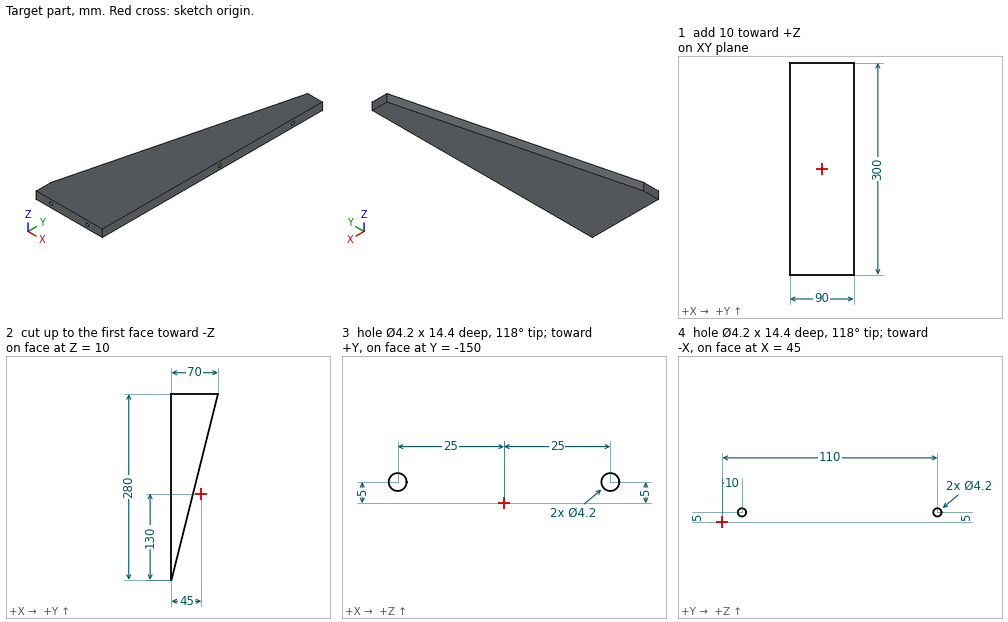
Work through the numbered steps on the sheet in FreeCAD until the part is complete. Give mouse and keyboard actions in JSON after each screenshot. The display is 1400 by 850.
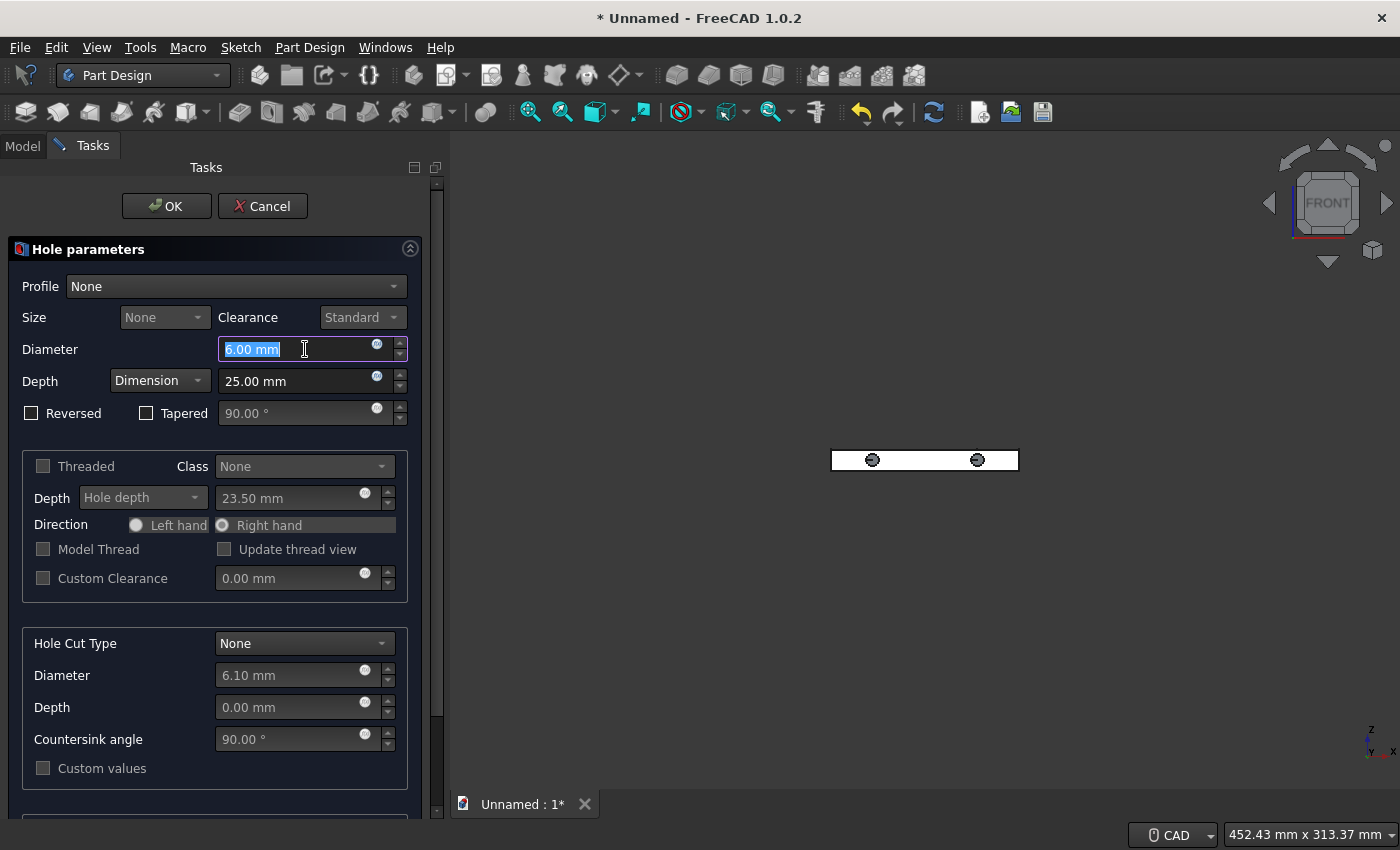
{"action": "type", "text": "4.2"}
{"action": "key", "text": "Tab"}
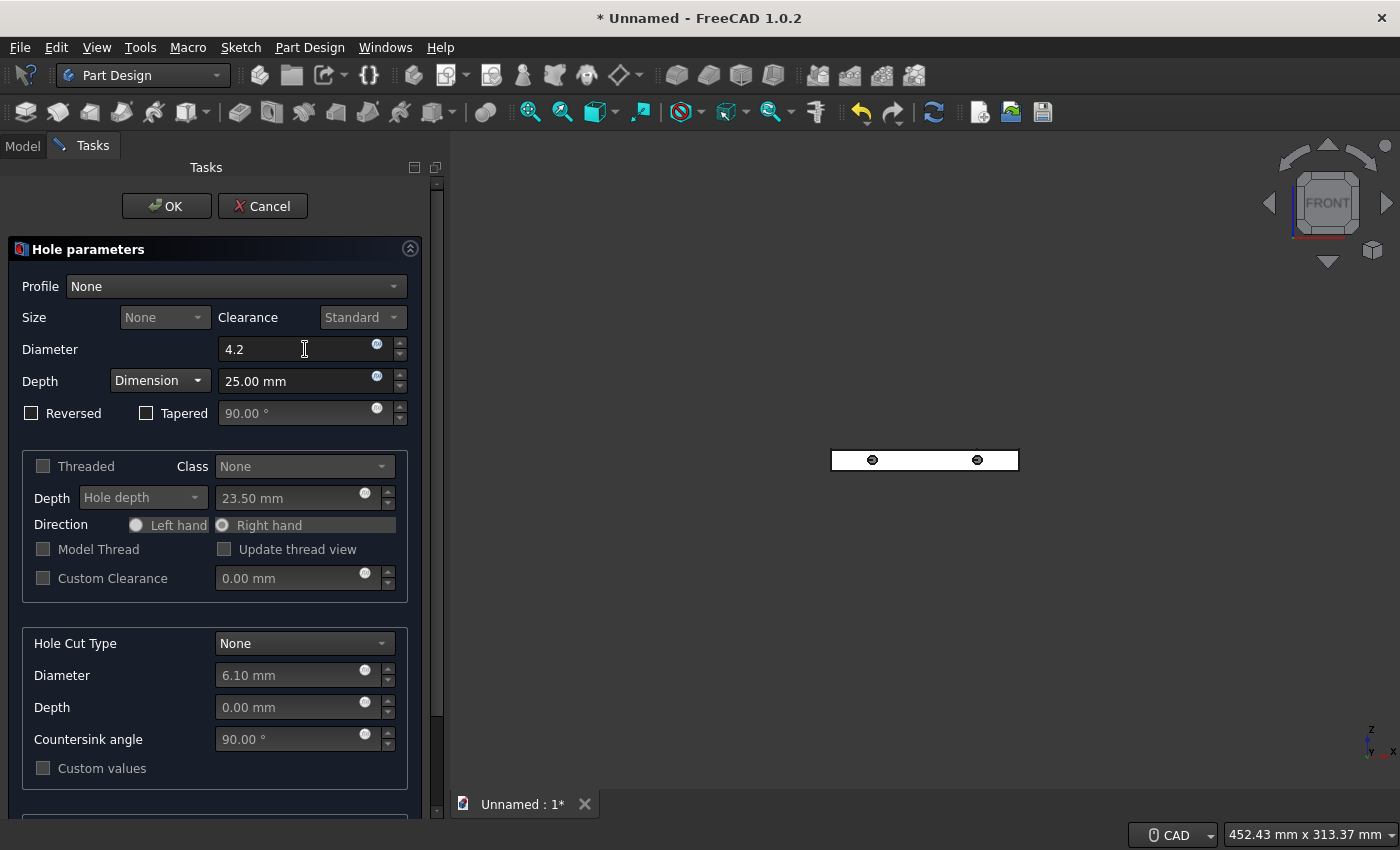
{"action": "triple_click", "coordinate": [305, 381]}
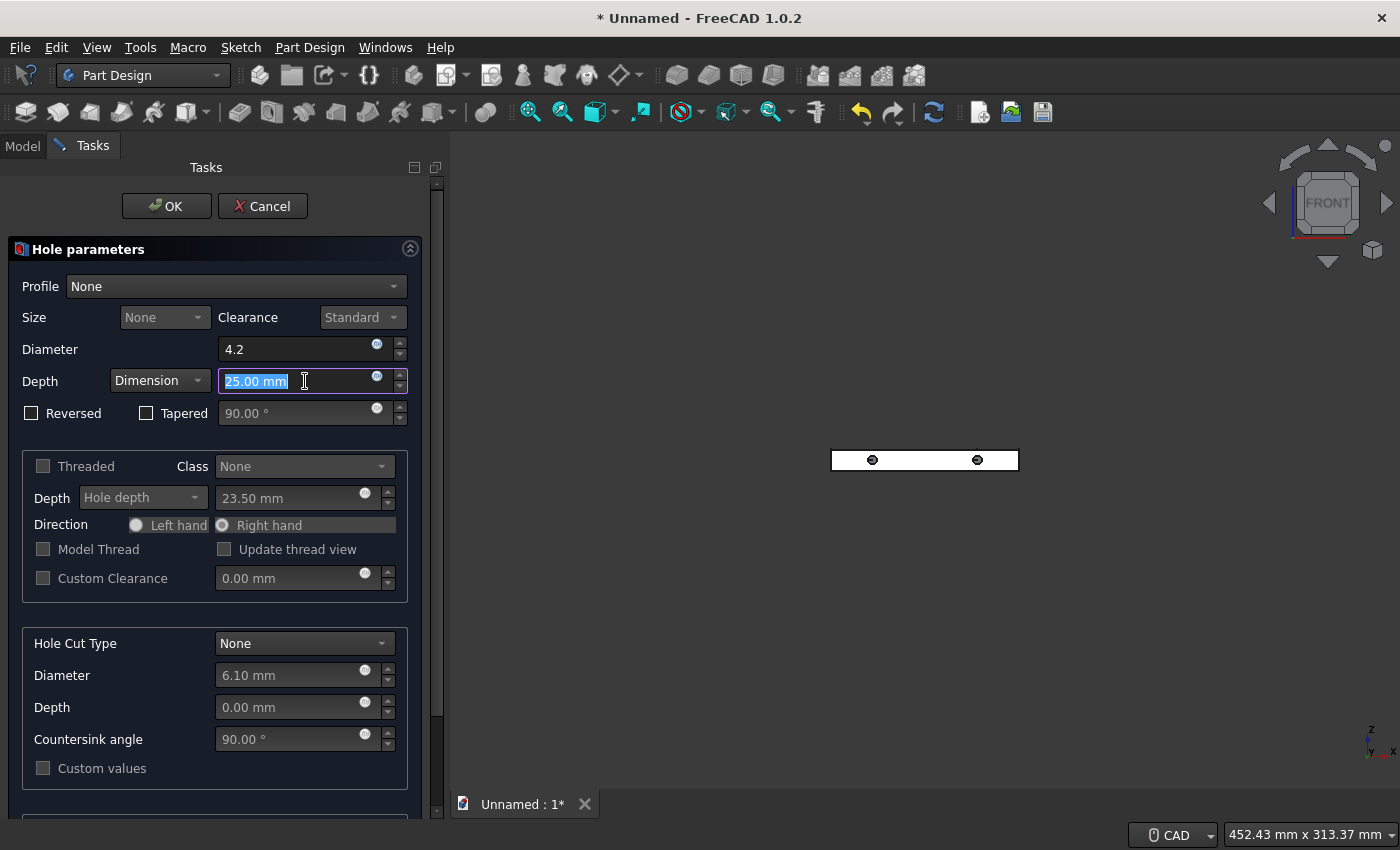
{"action": "type", "text": "14.4"}
{"action": "key", "text": "Tab"}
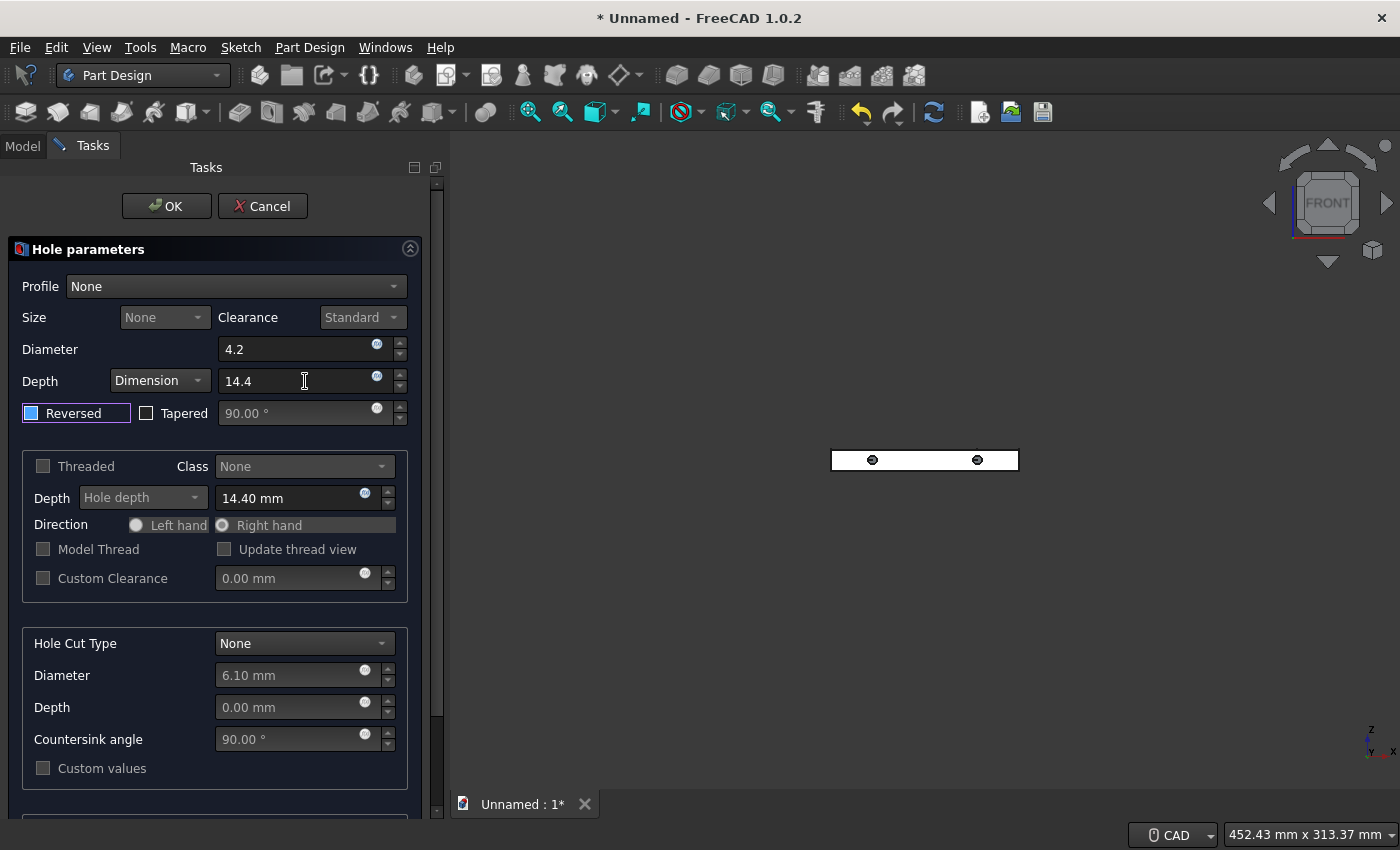
{"action": "left_click", "coordinate": [167, 206]}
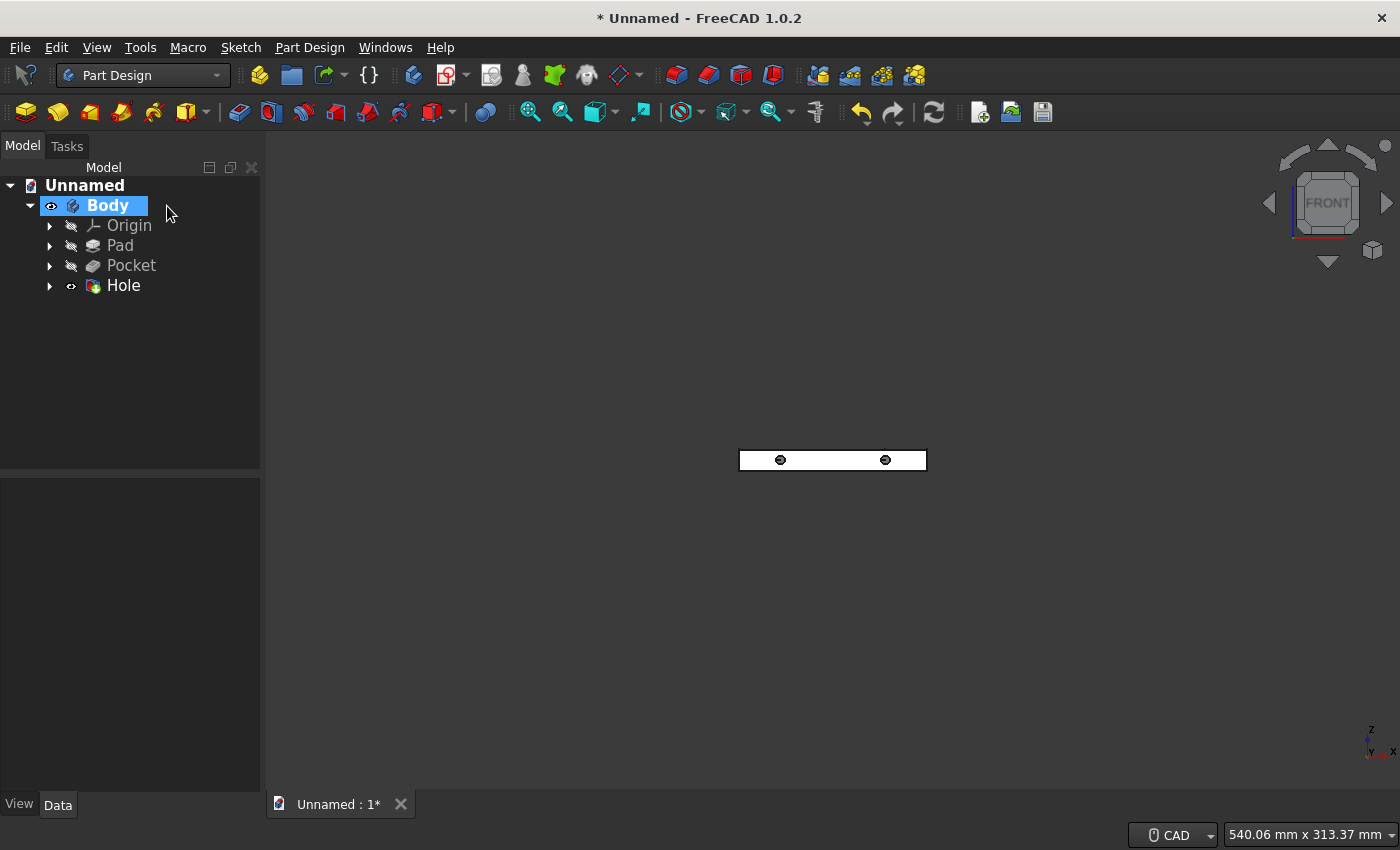
{"action": "key", "text": "v f"}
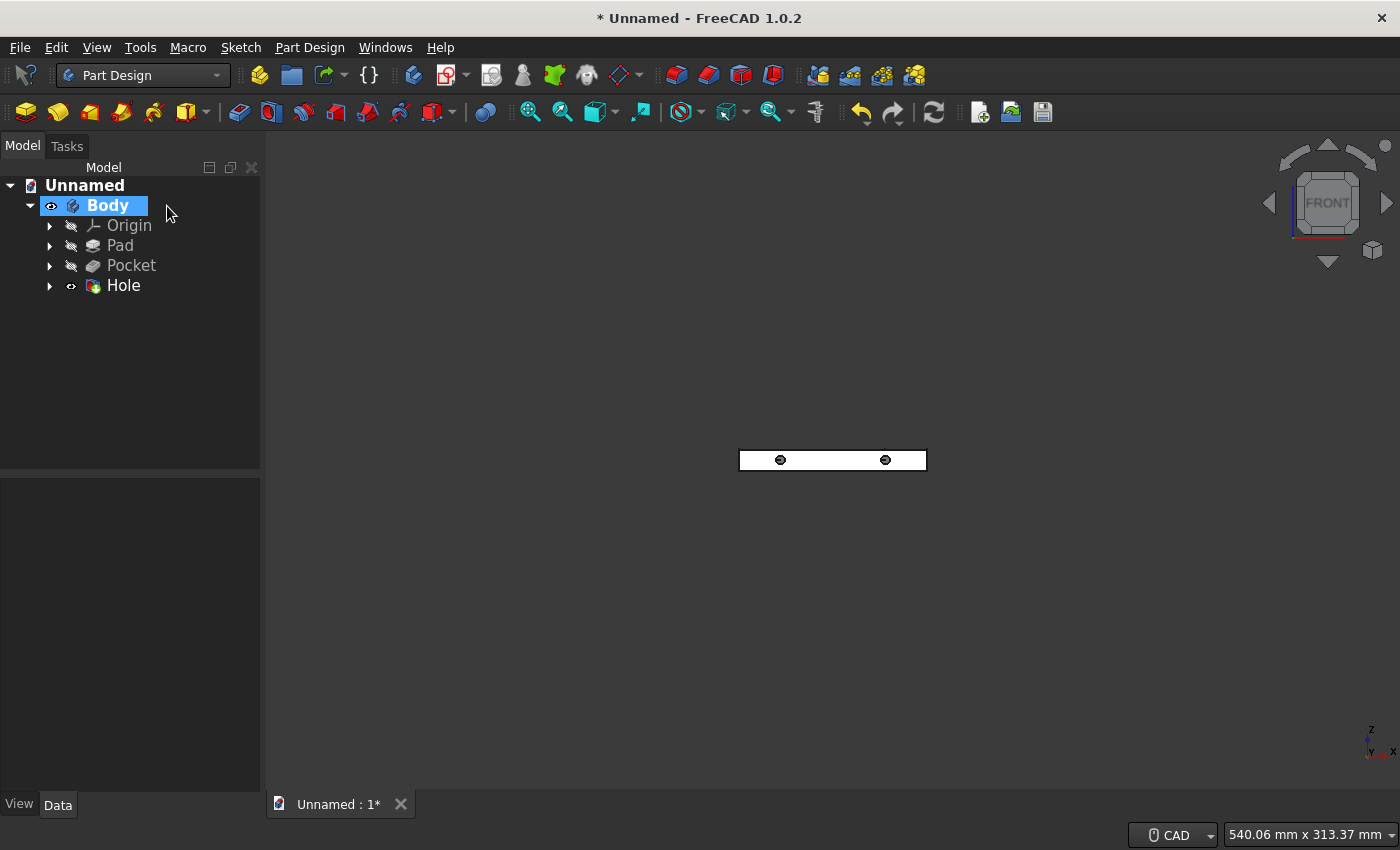
{"action": "key", "text": "0"}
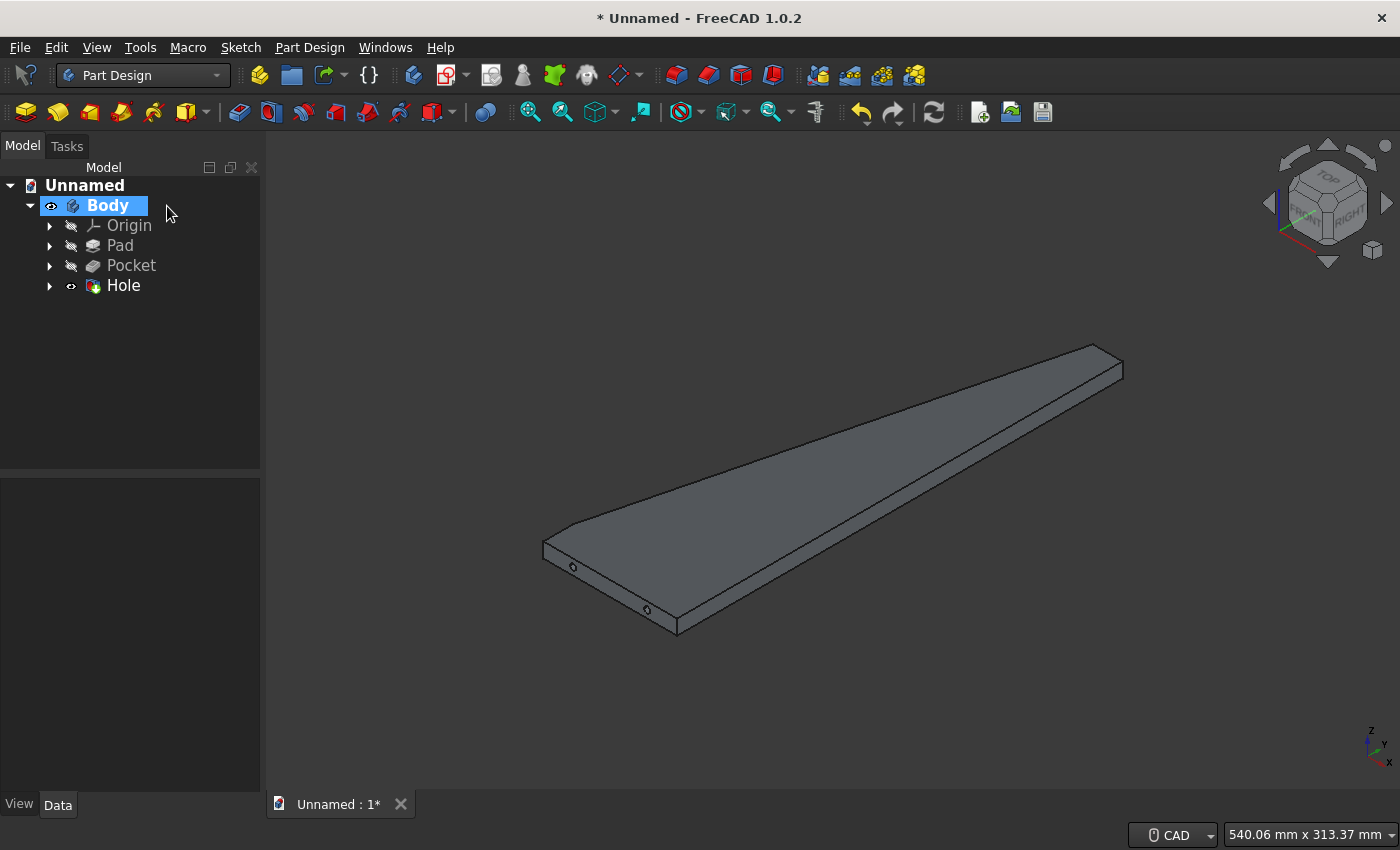
{"action": "key", "text": "3"}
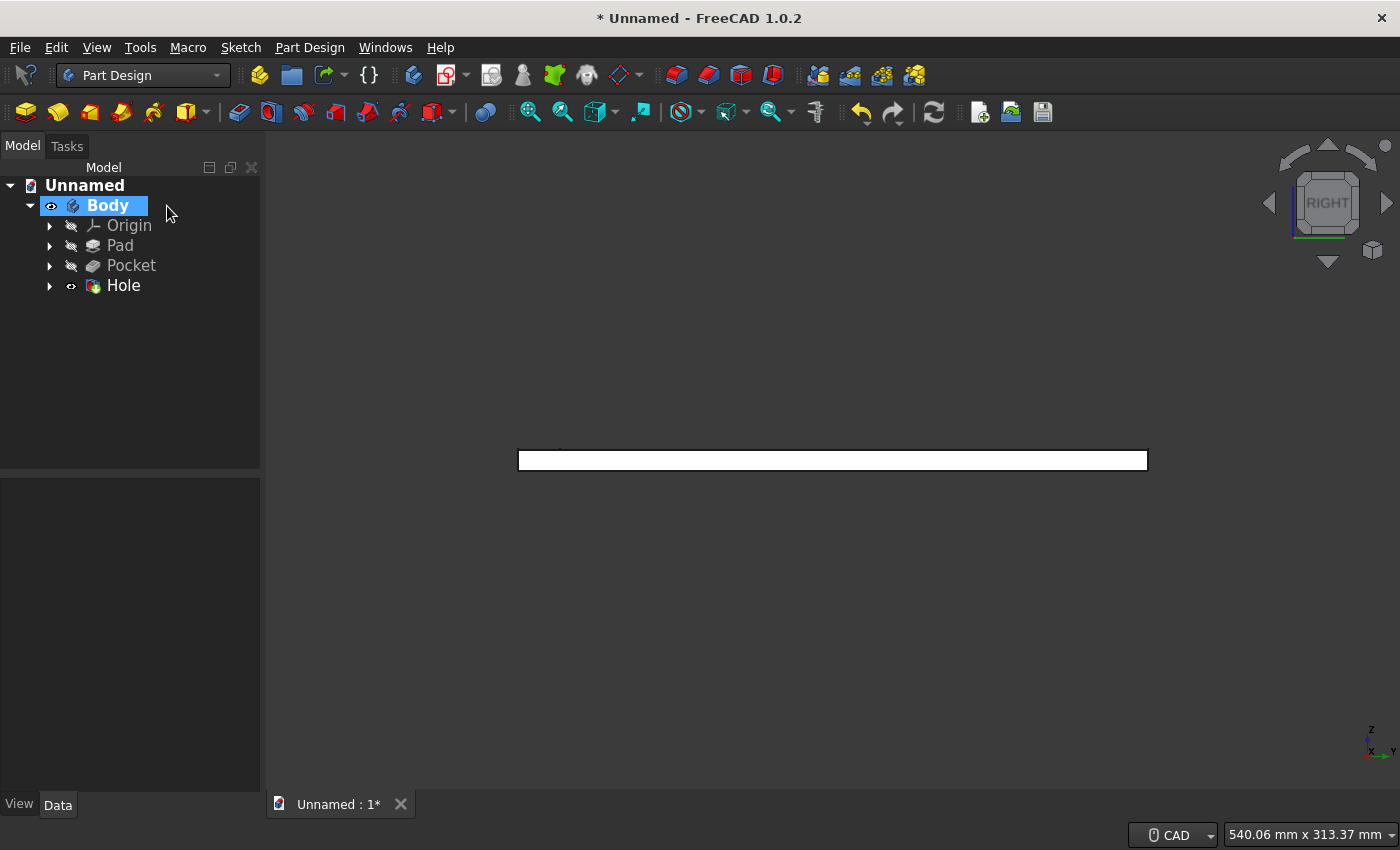
{"action": "left_click", "coordinate": [1103, 459]}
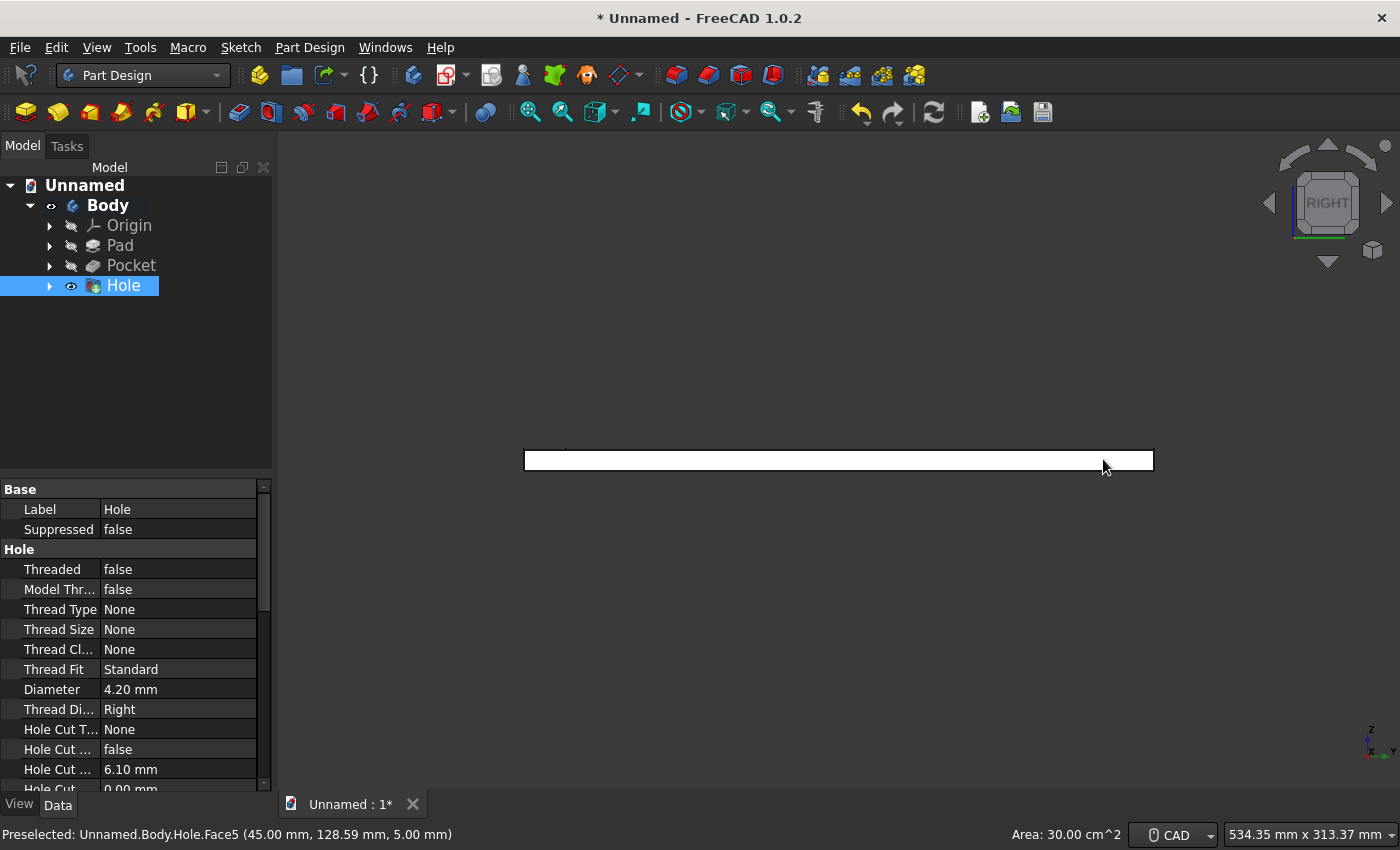
{"action": "left_click", "coordinate": [446, 76]}